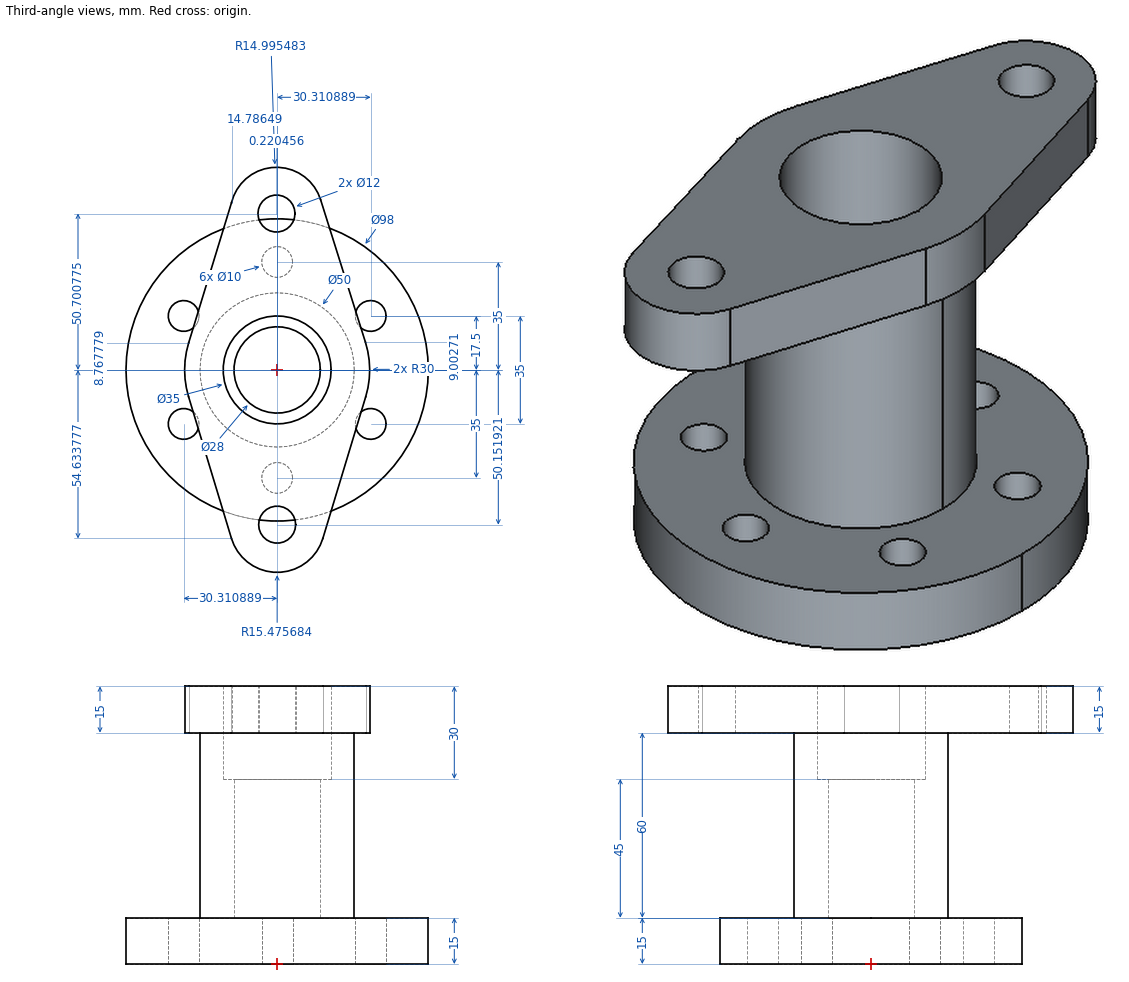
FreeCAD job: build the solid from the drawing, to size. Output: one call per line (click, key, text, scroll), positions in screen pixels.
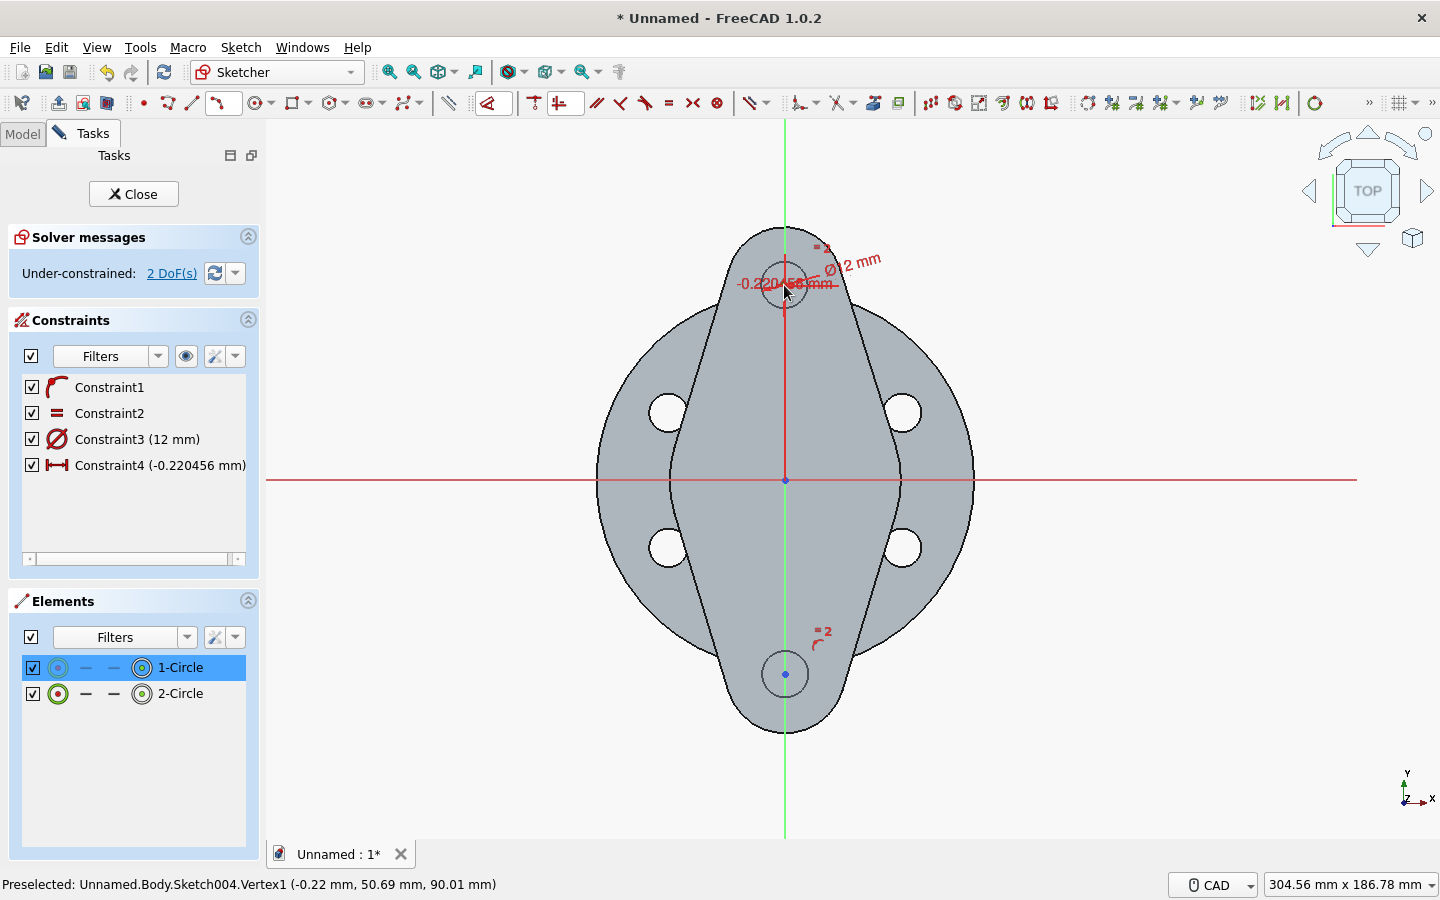
key(i)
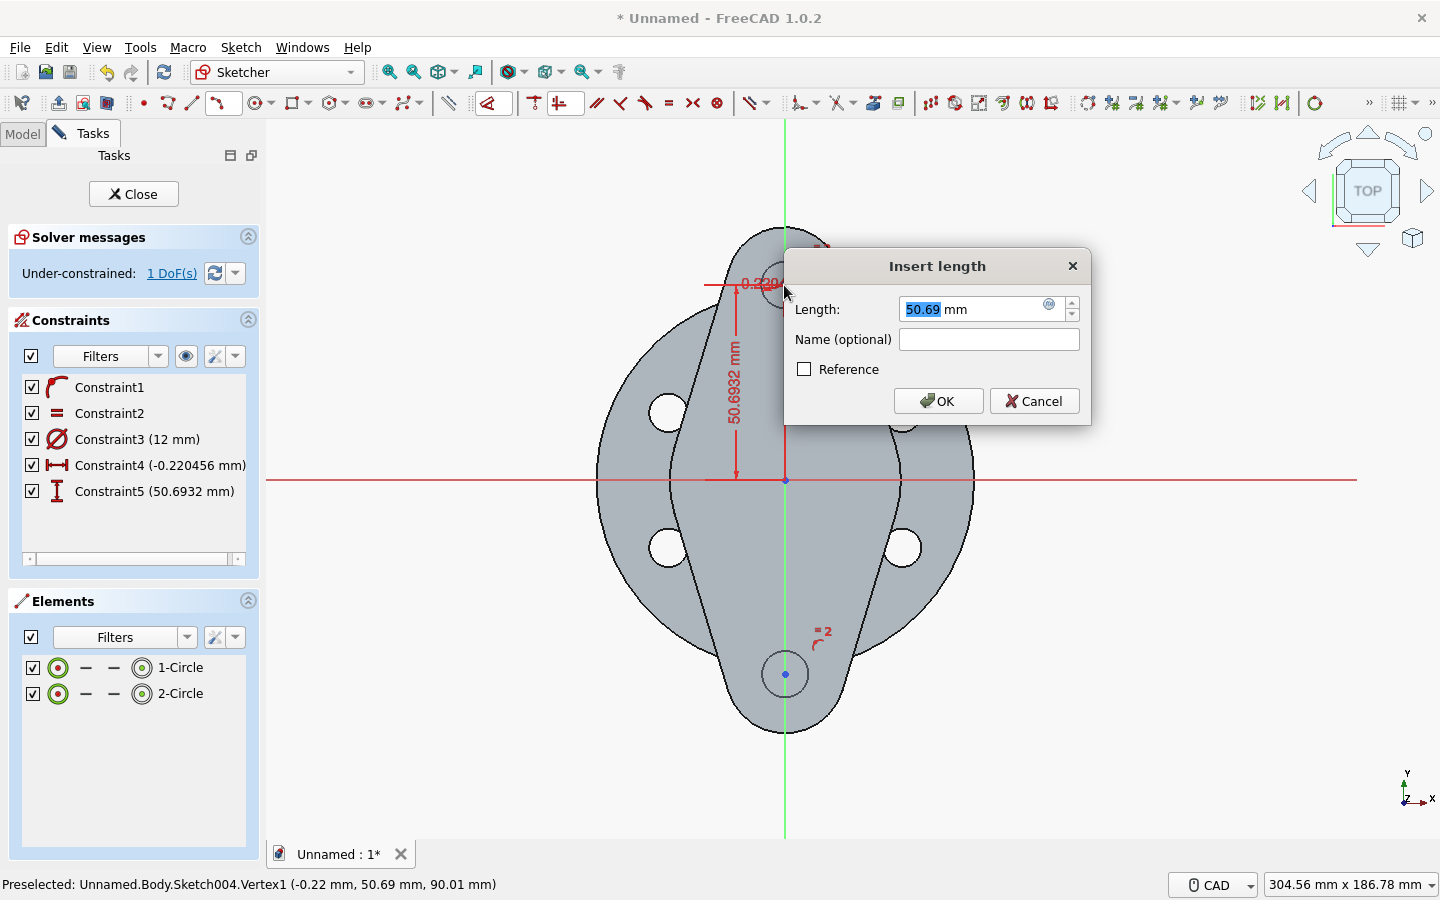
text(50.700775)
key(Return)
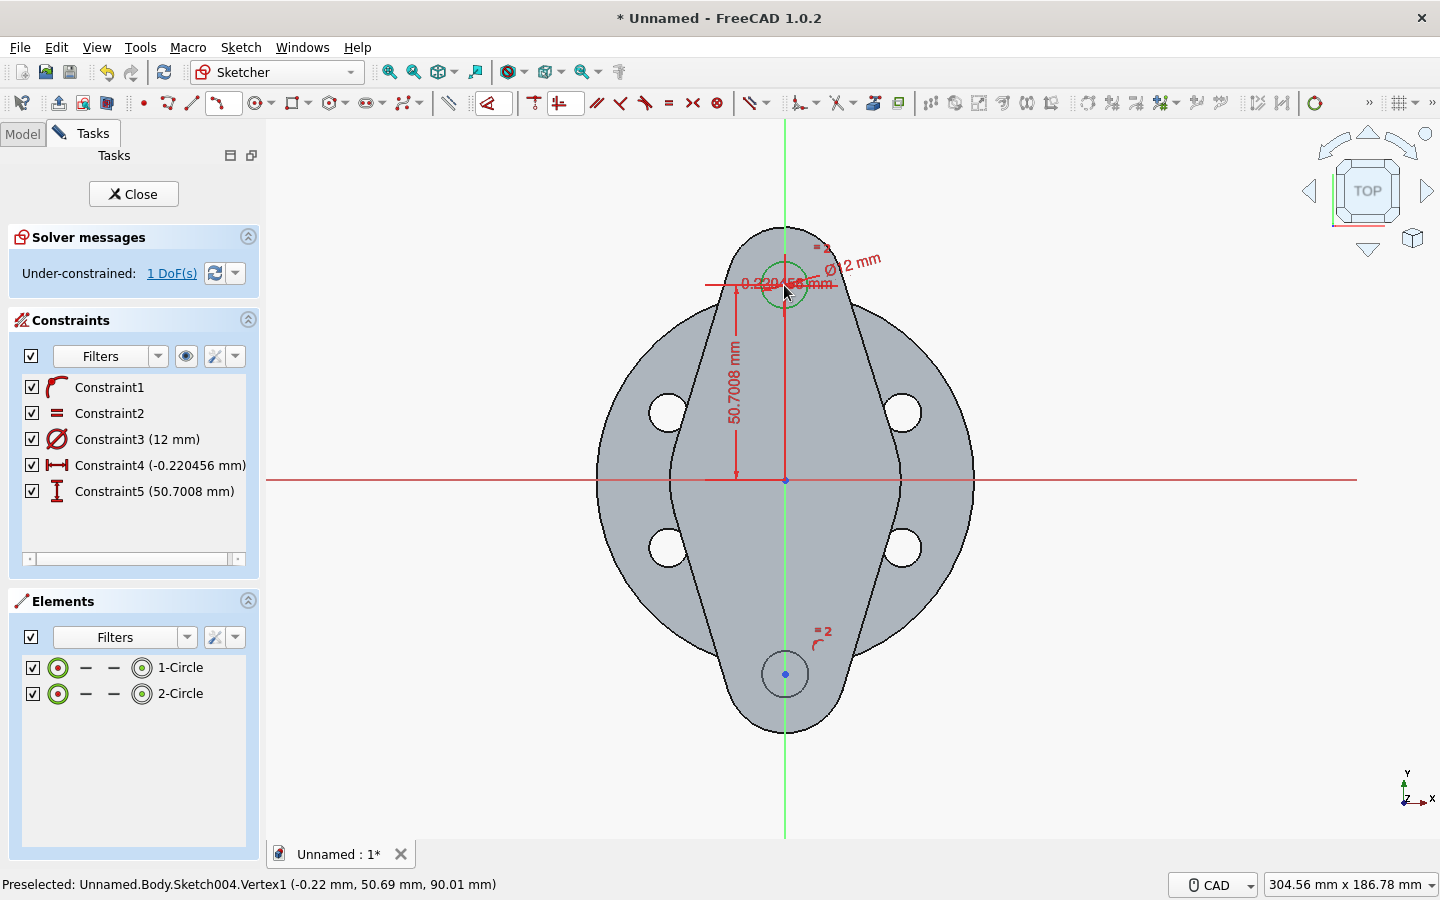
click(785, 674)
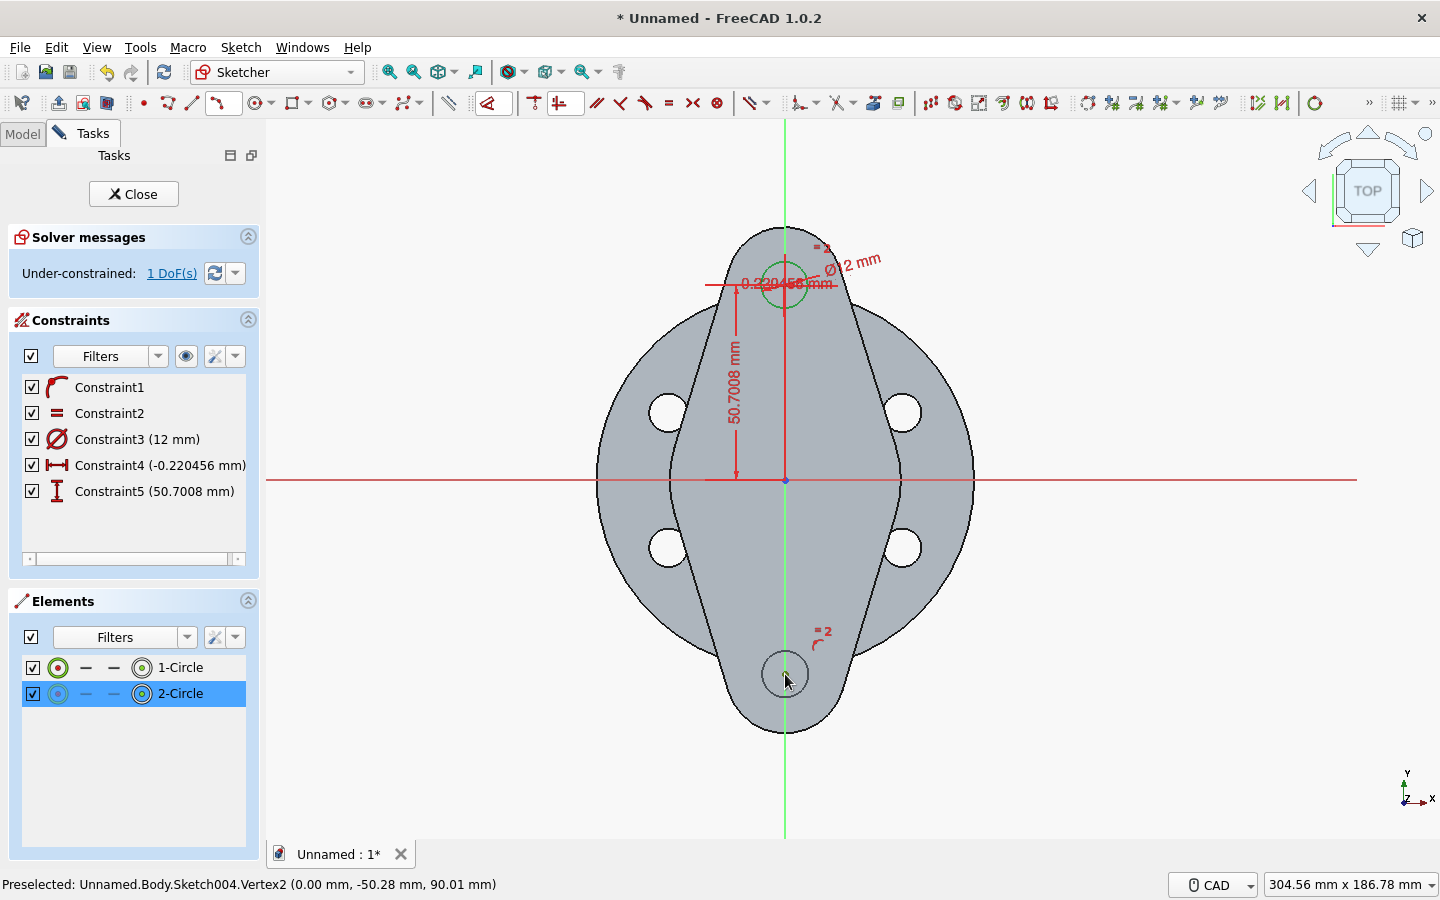
key(i)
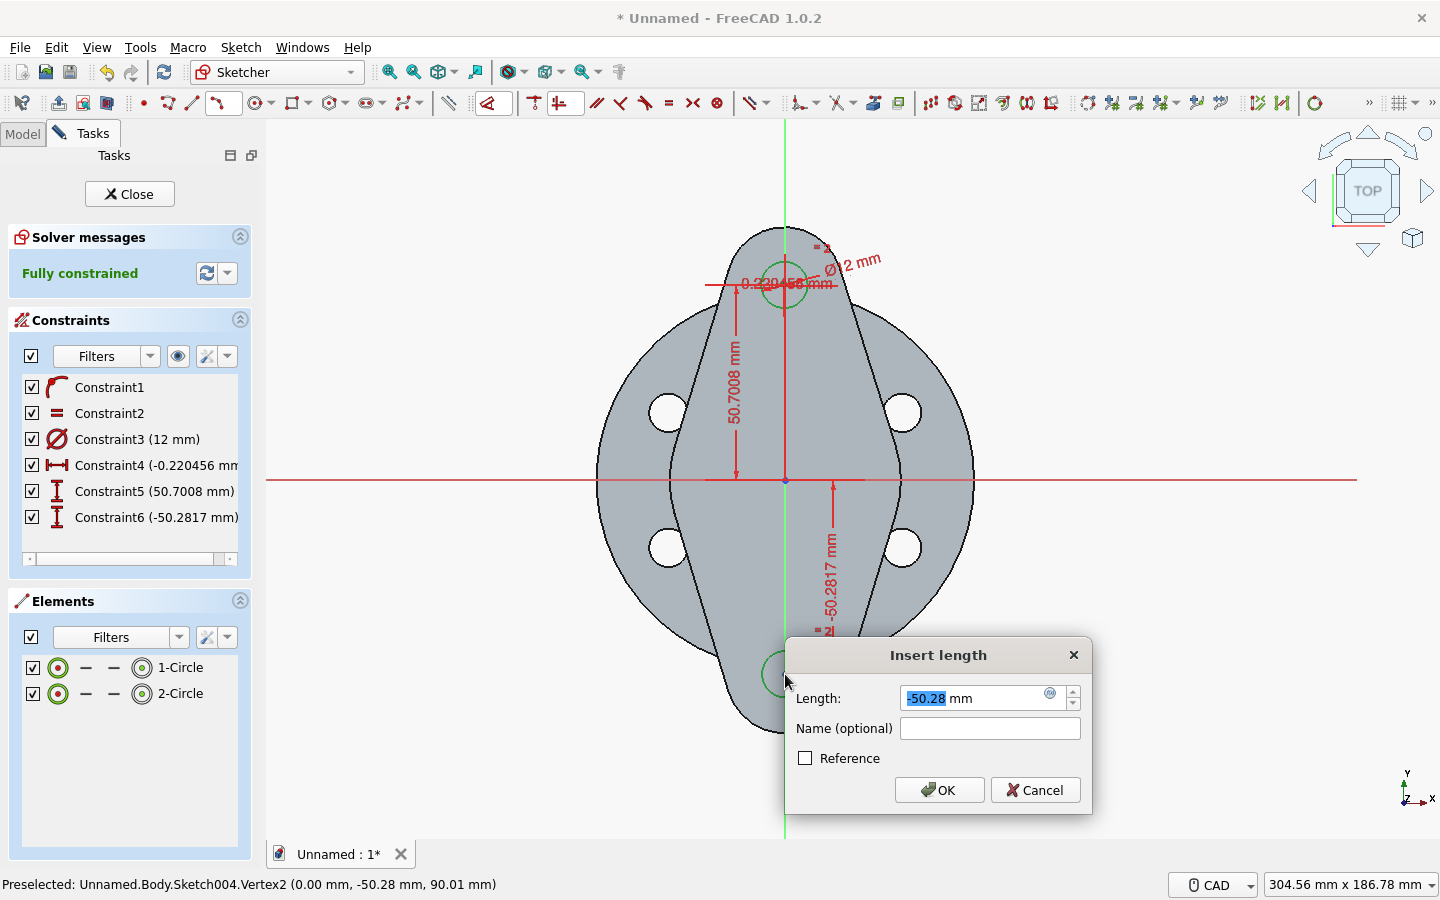
text(-50.151921)
key(Return)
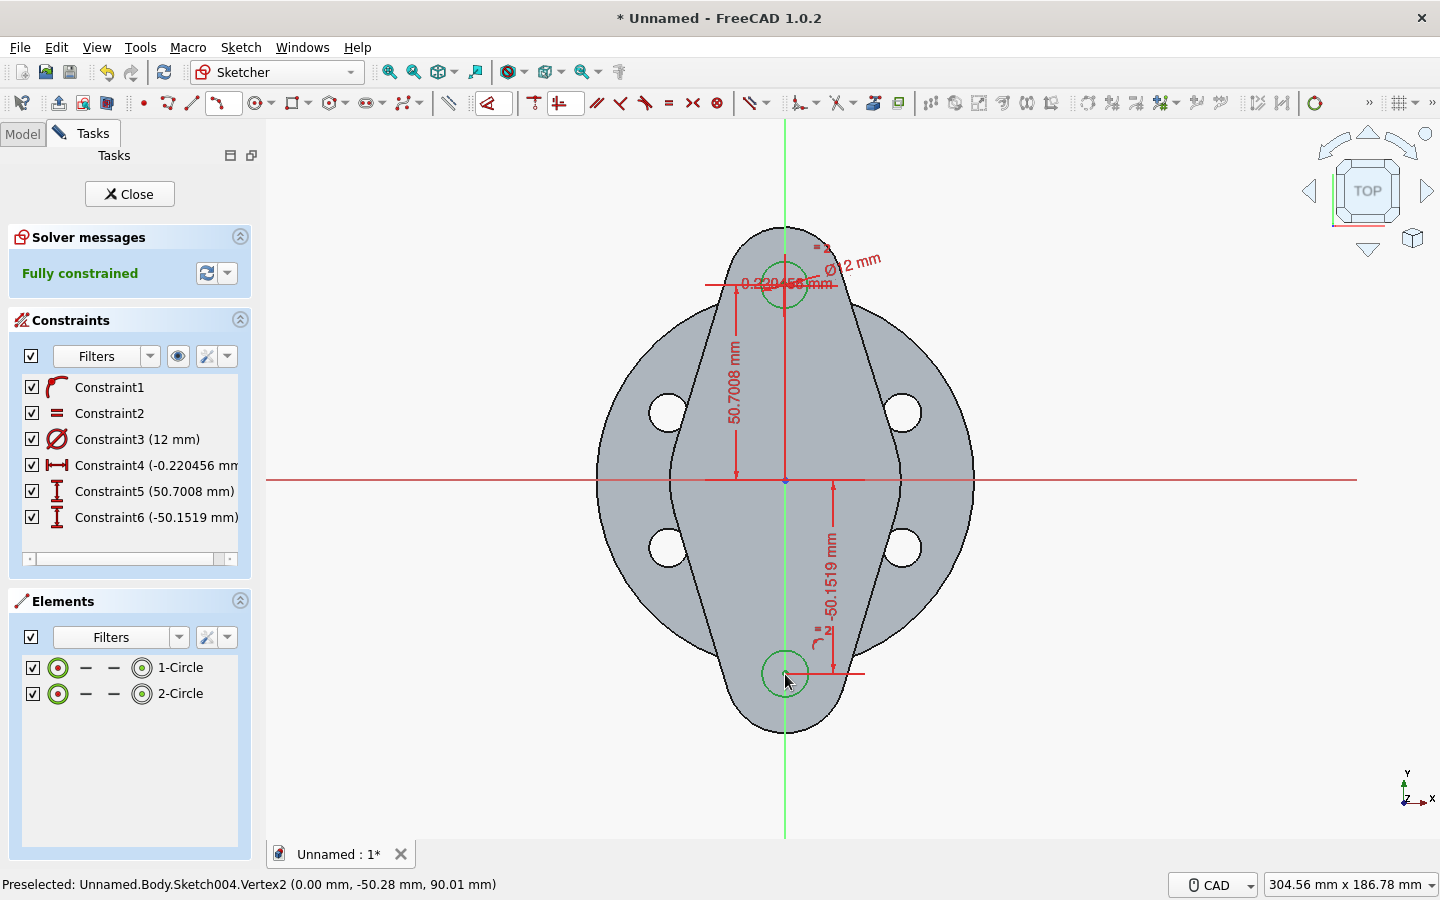
click(130, 194)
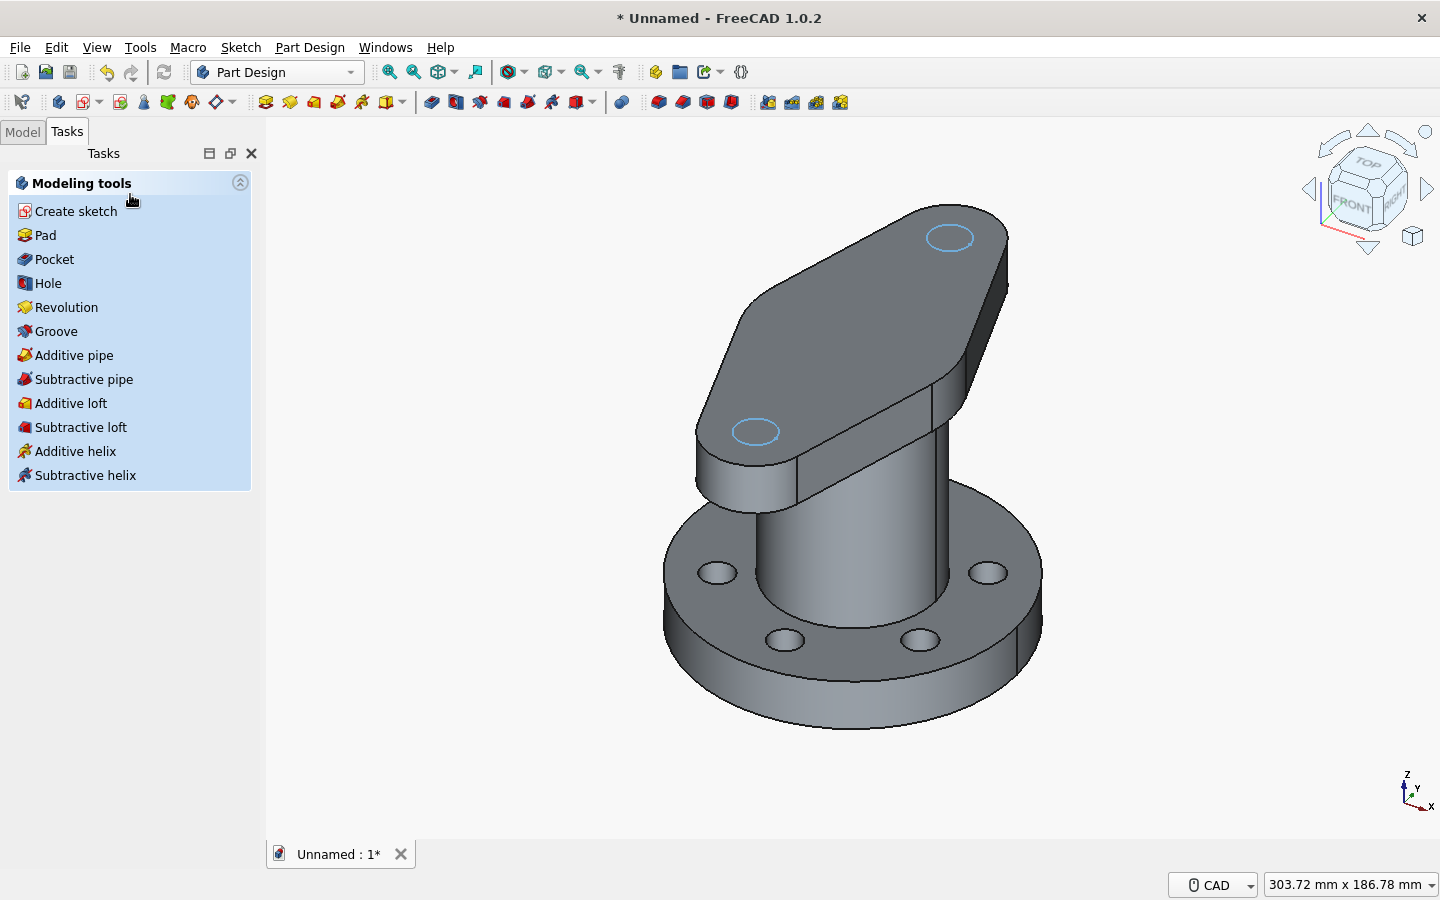
click(432, 102)